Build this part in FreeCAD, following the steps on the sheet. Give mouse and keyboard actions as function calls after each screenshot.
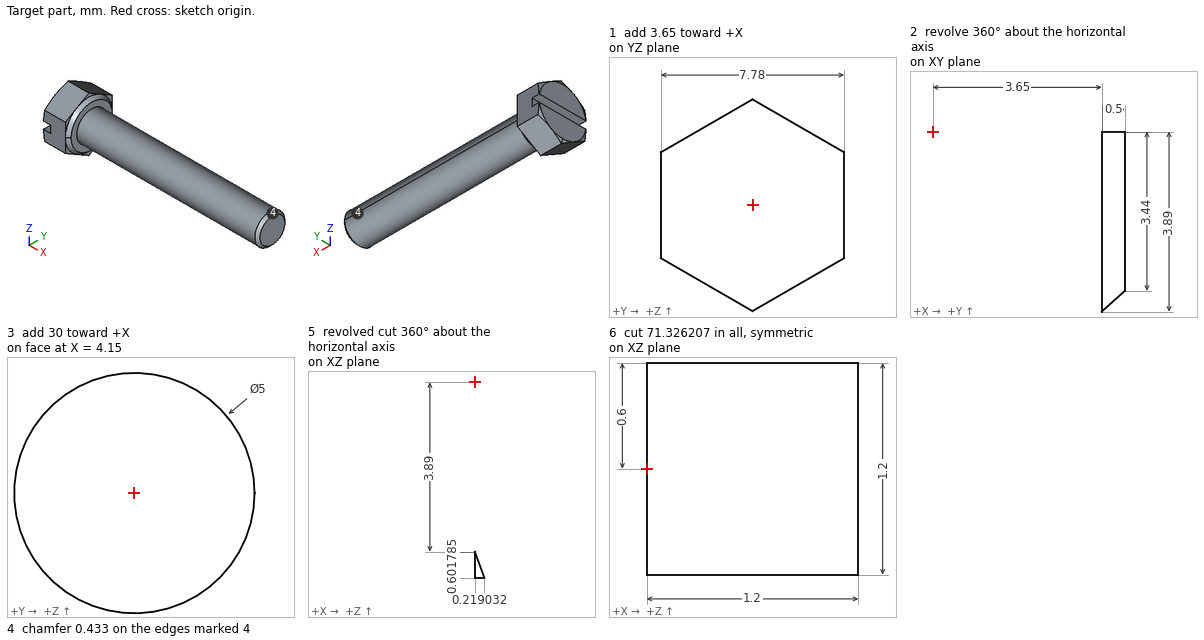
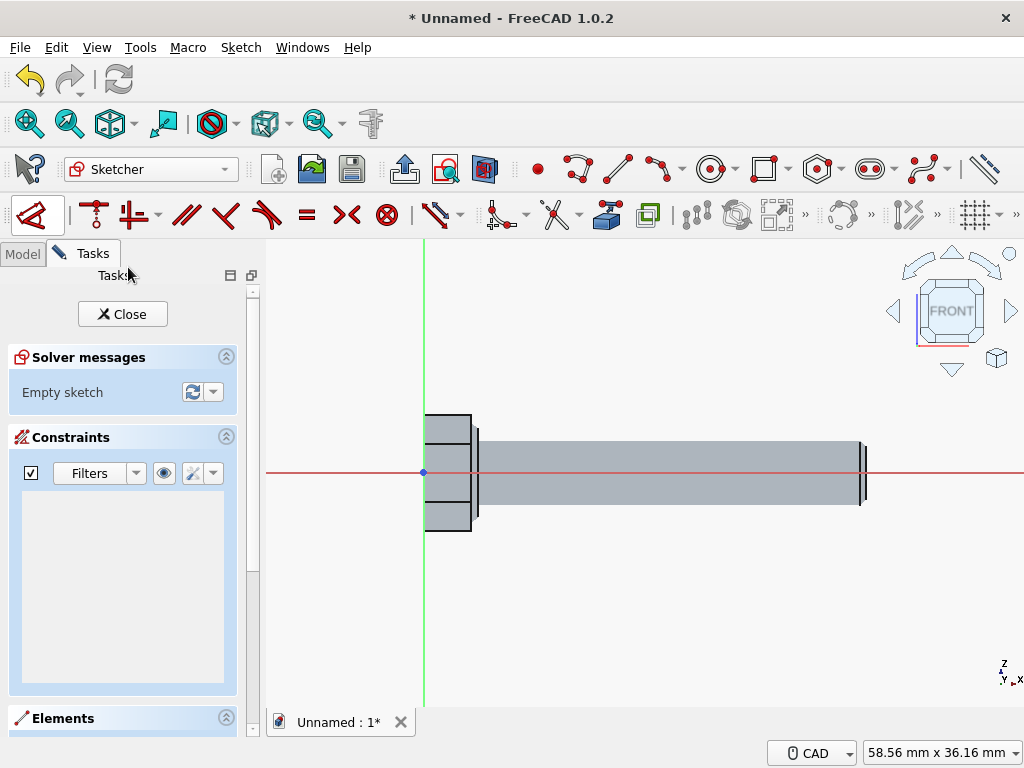
scroll(418, 530, up, 15)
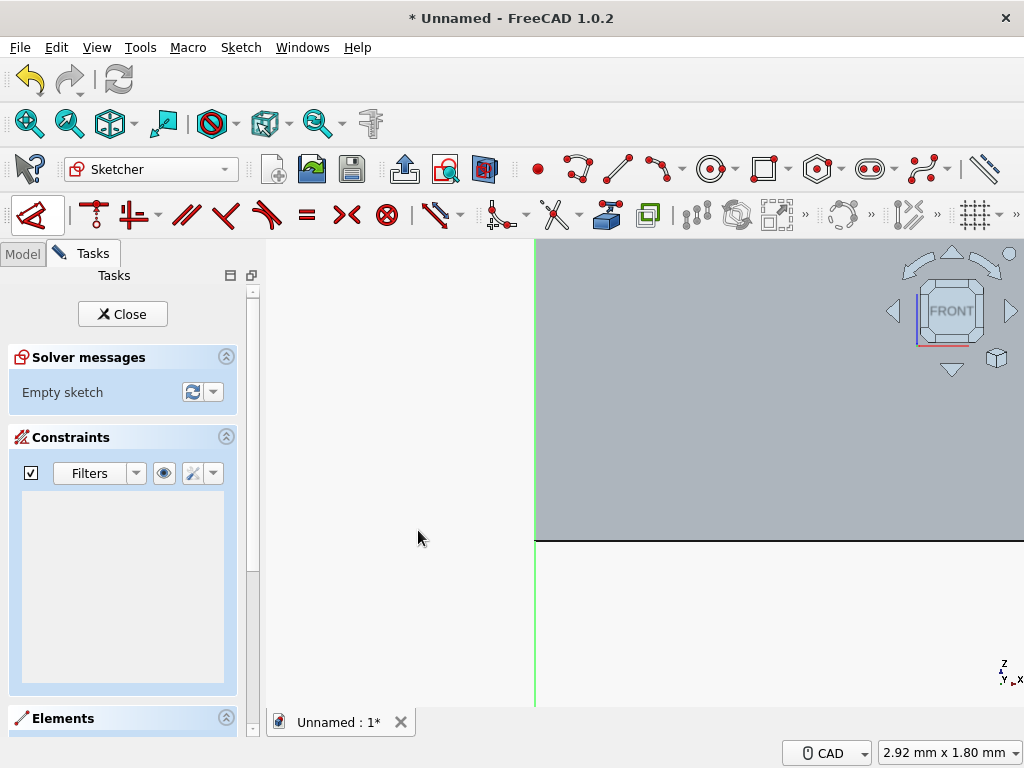
scroll(547, 450, up, 3)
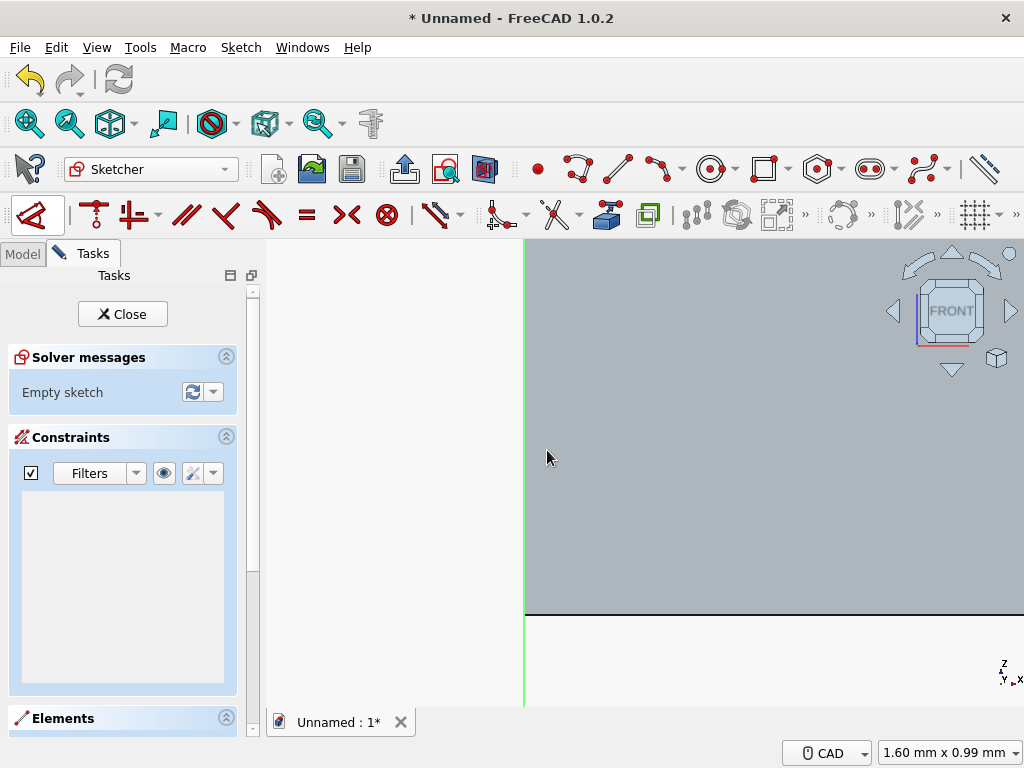
key(g)
key(m)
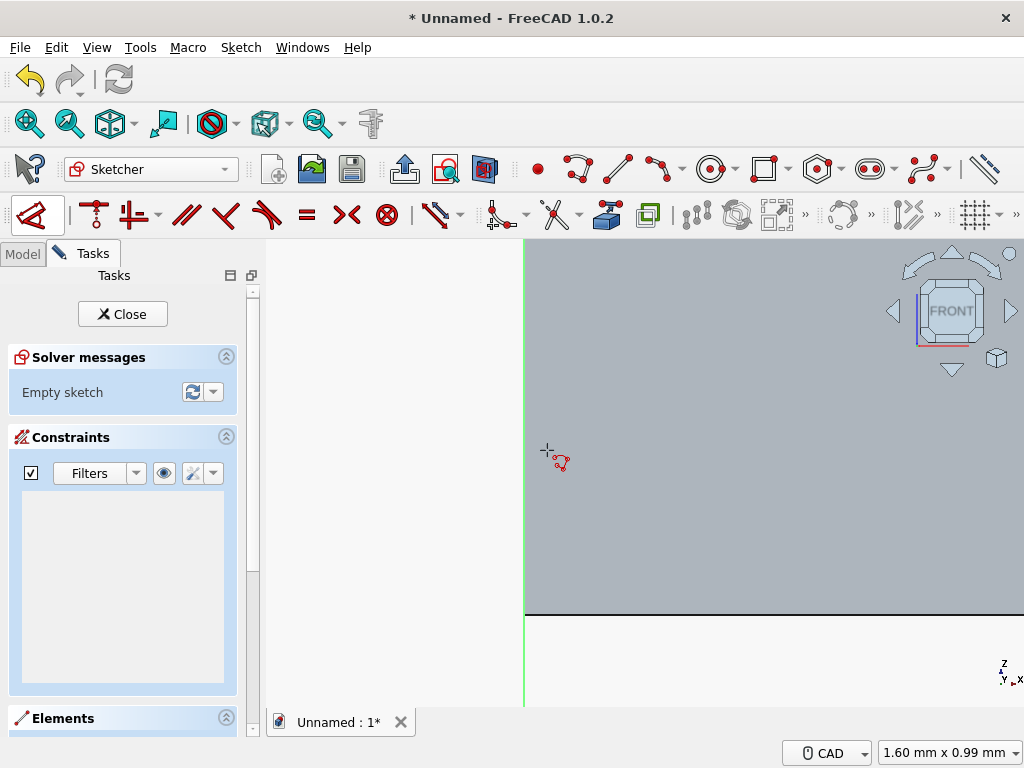
click(524, 330)
click(628, 615)
click(533, 615)
click(524, 331)
key(Escape)
key(Escape)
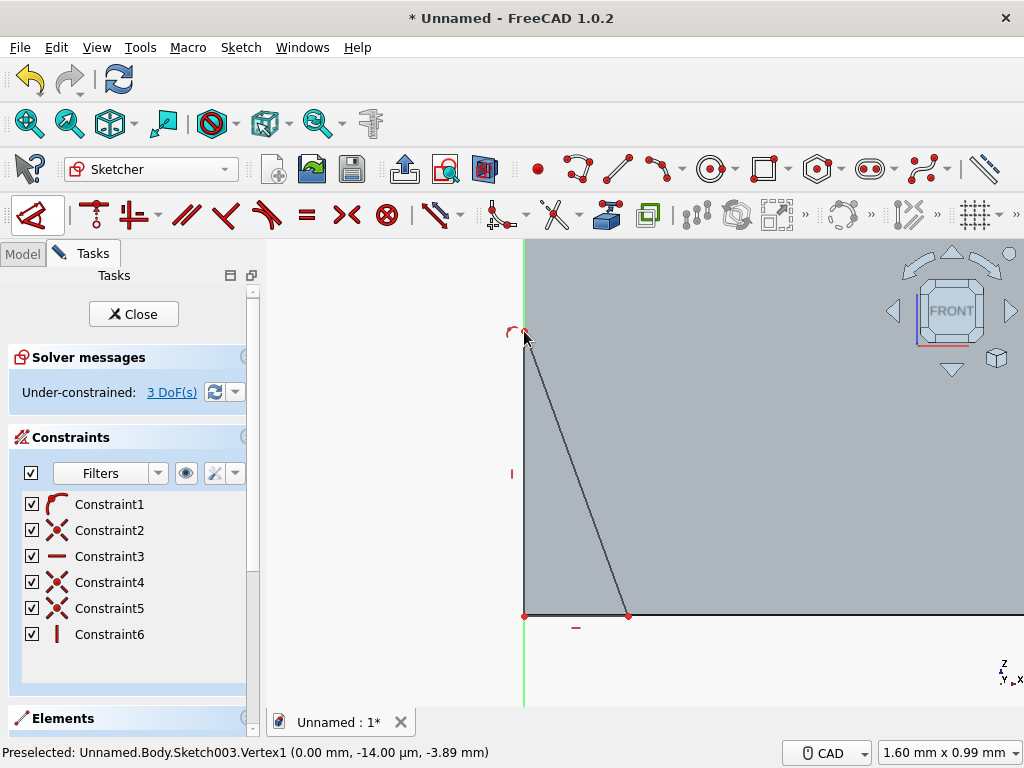
click(524, 331)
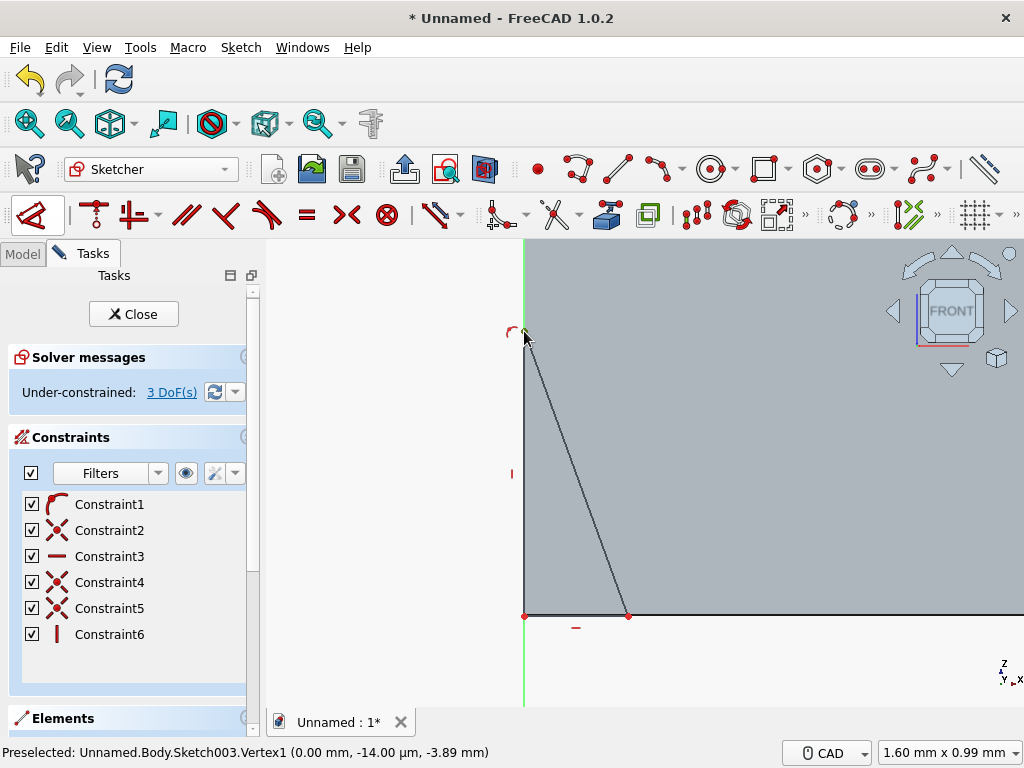
key(i)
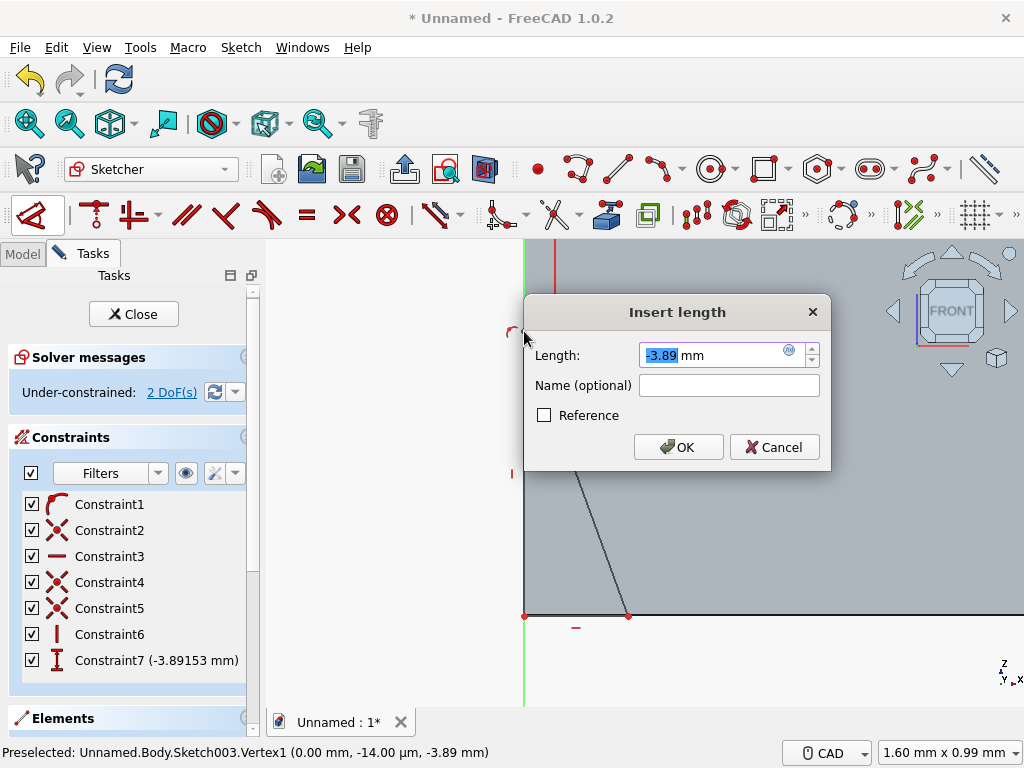
text(-3.89)
key(Return)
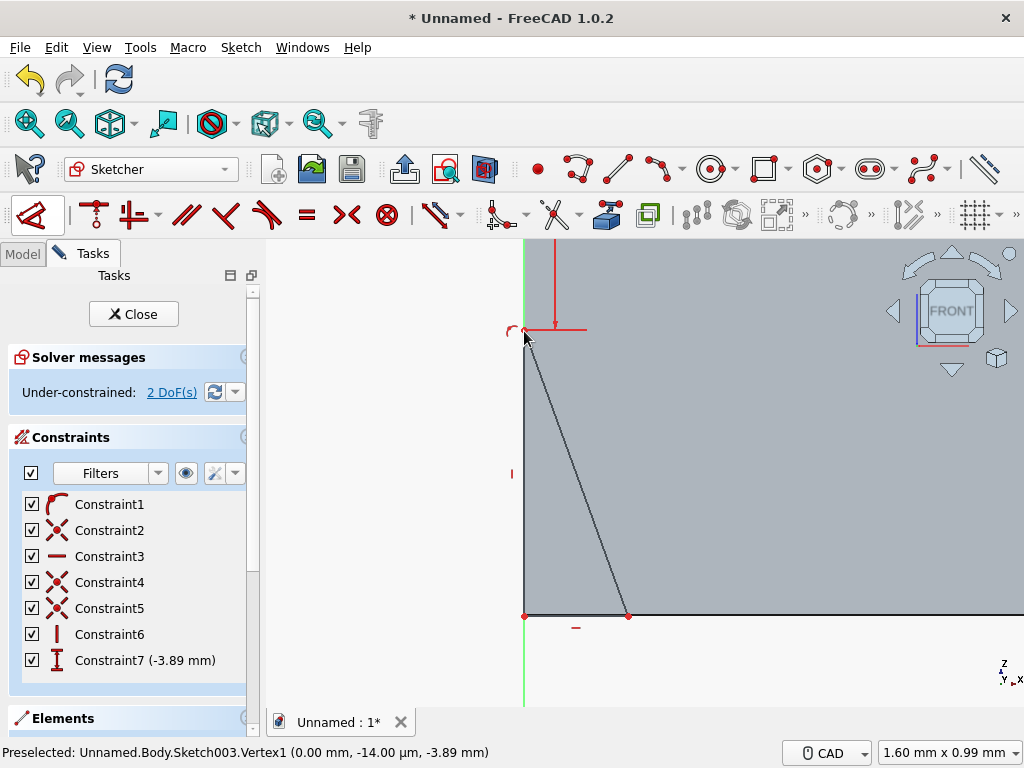
click(597, 616)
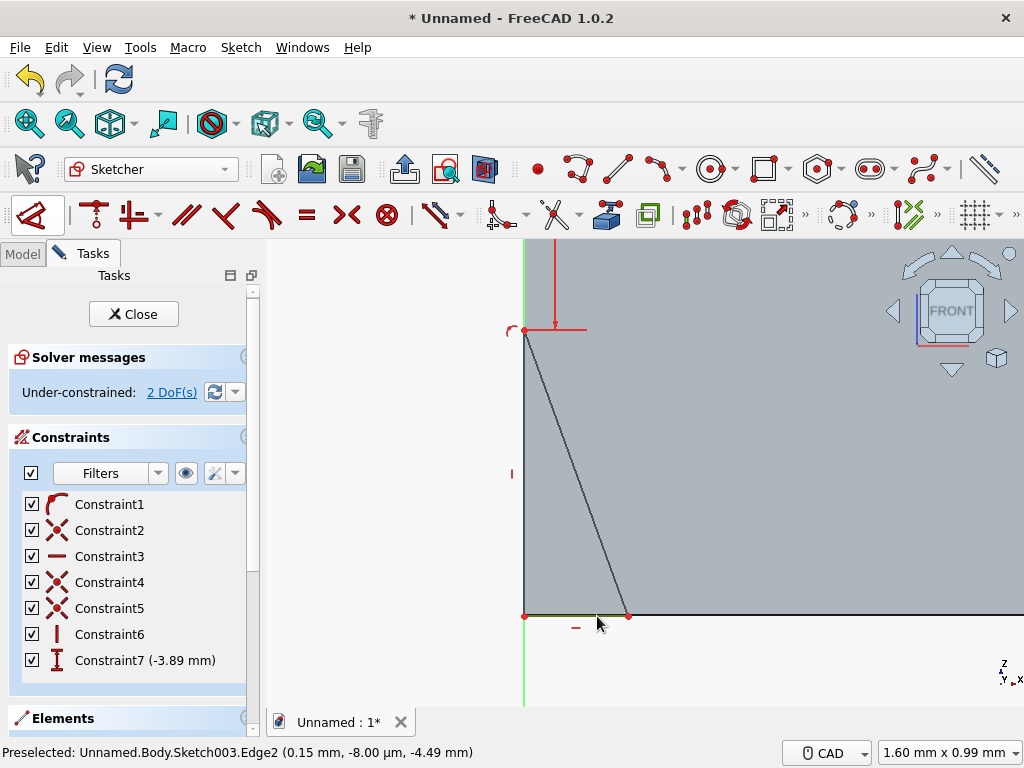
key(l)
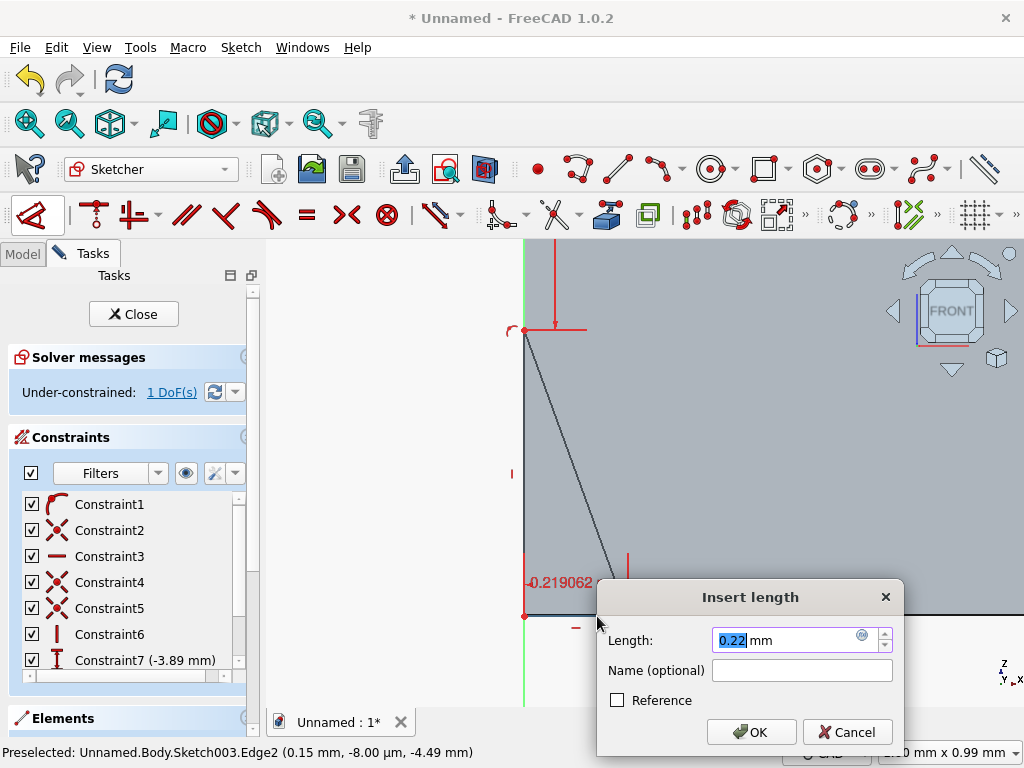
text(0.219032)
key(Return)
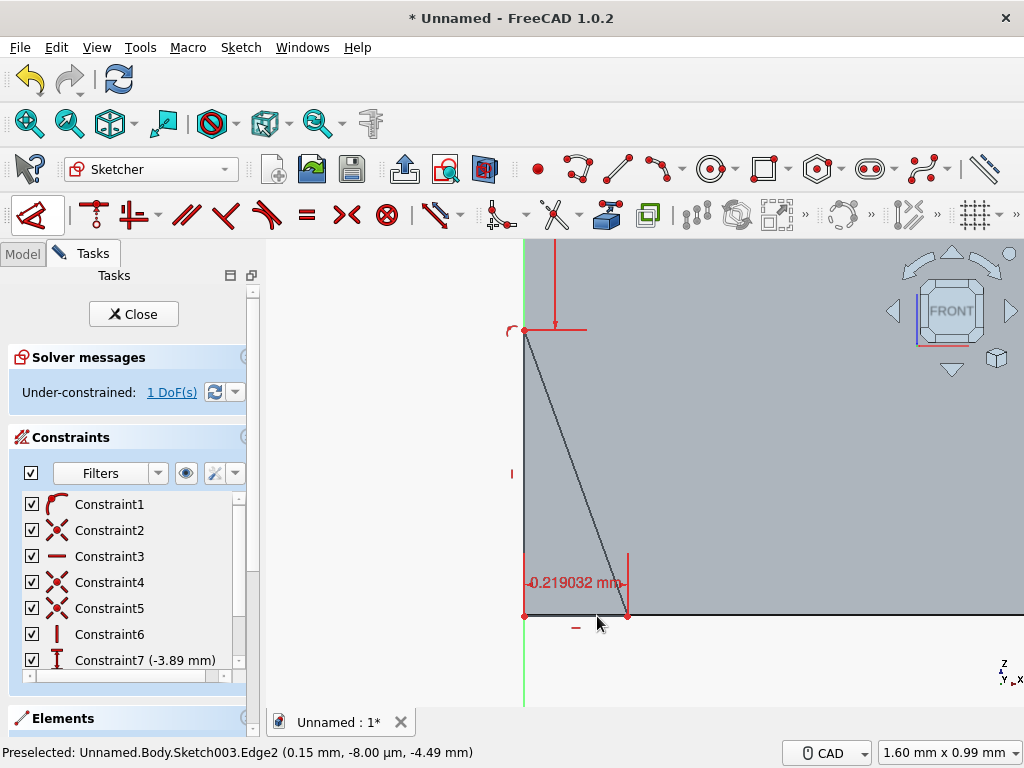
click(524, 530)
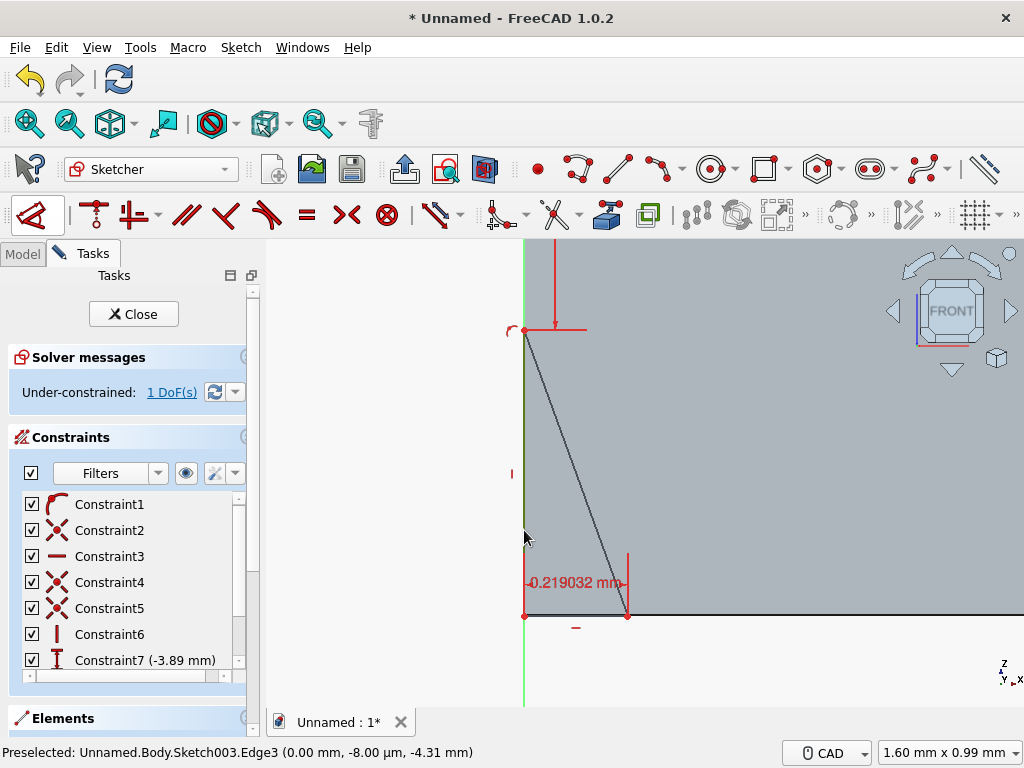
key(i)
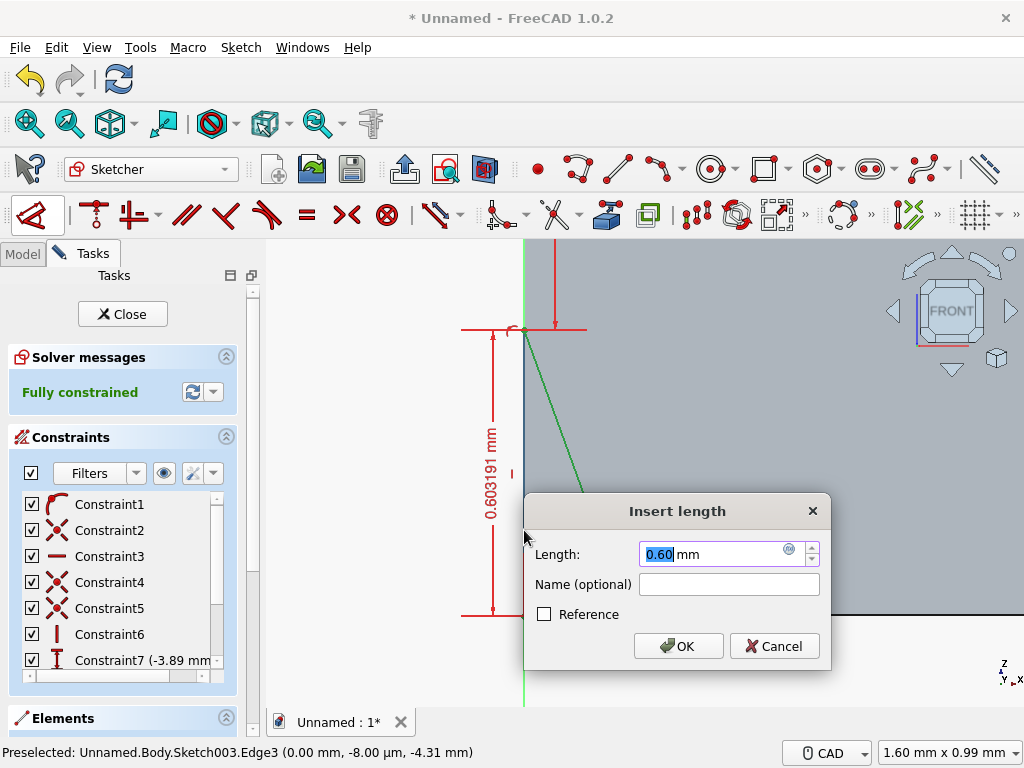
text(0.601785)
key(Return)